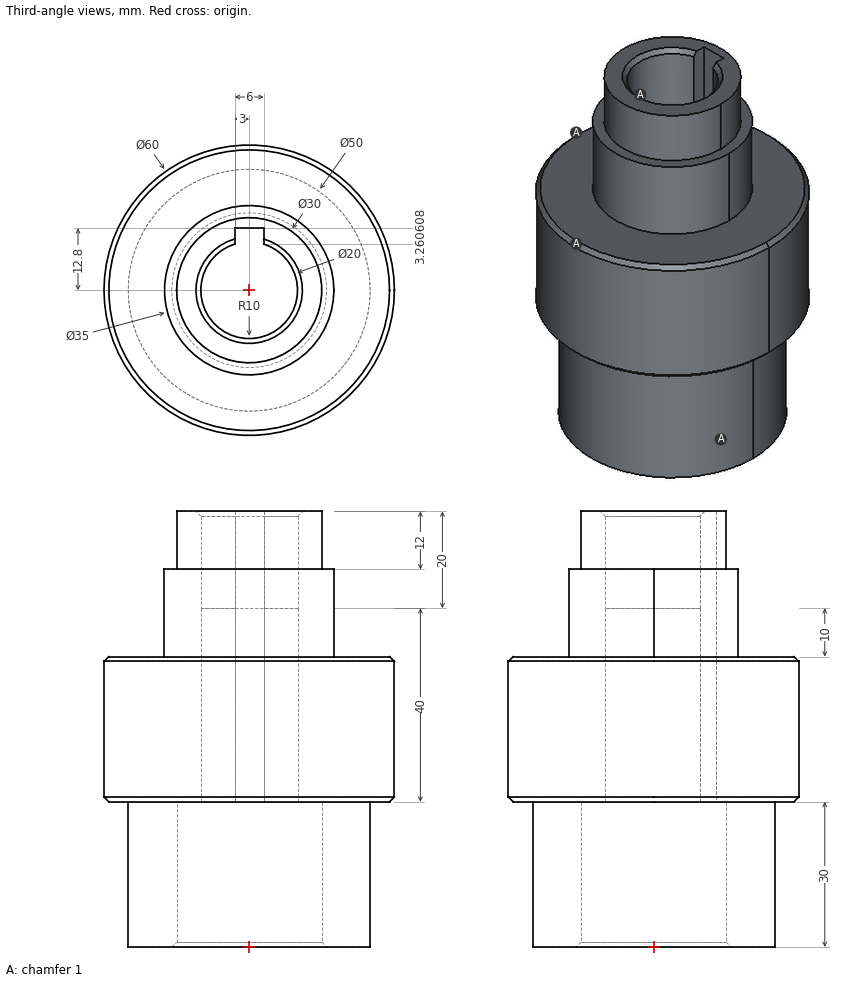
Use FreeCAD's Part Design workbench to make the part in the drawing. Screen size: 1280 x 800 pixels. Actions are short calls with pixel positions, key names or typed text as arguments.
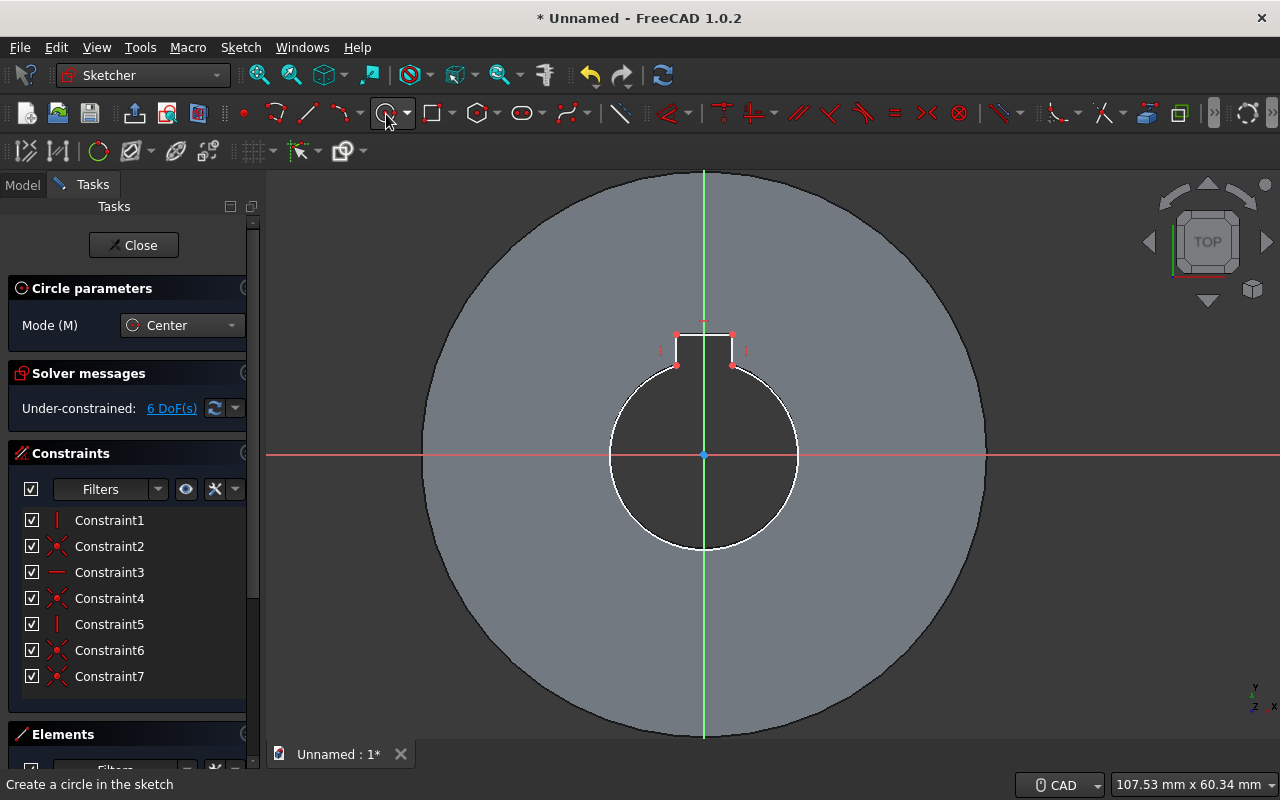
click(704, 454)
move(821, 338)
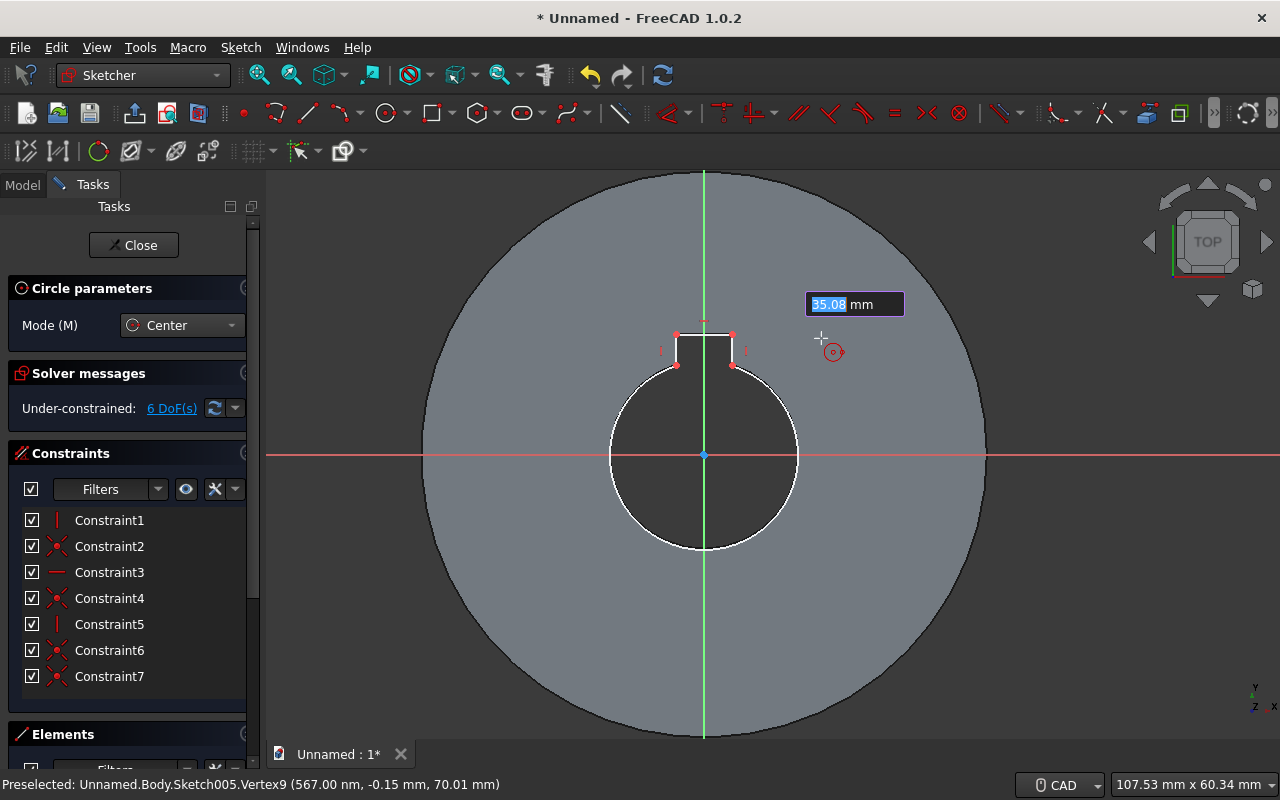
text(35)
key(Return)
key(Escape)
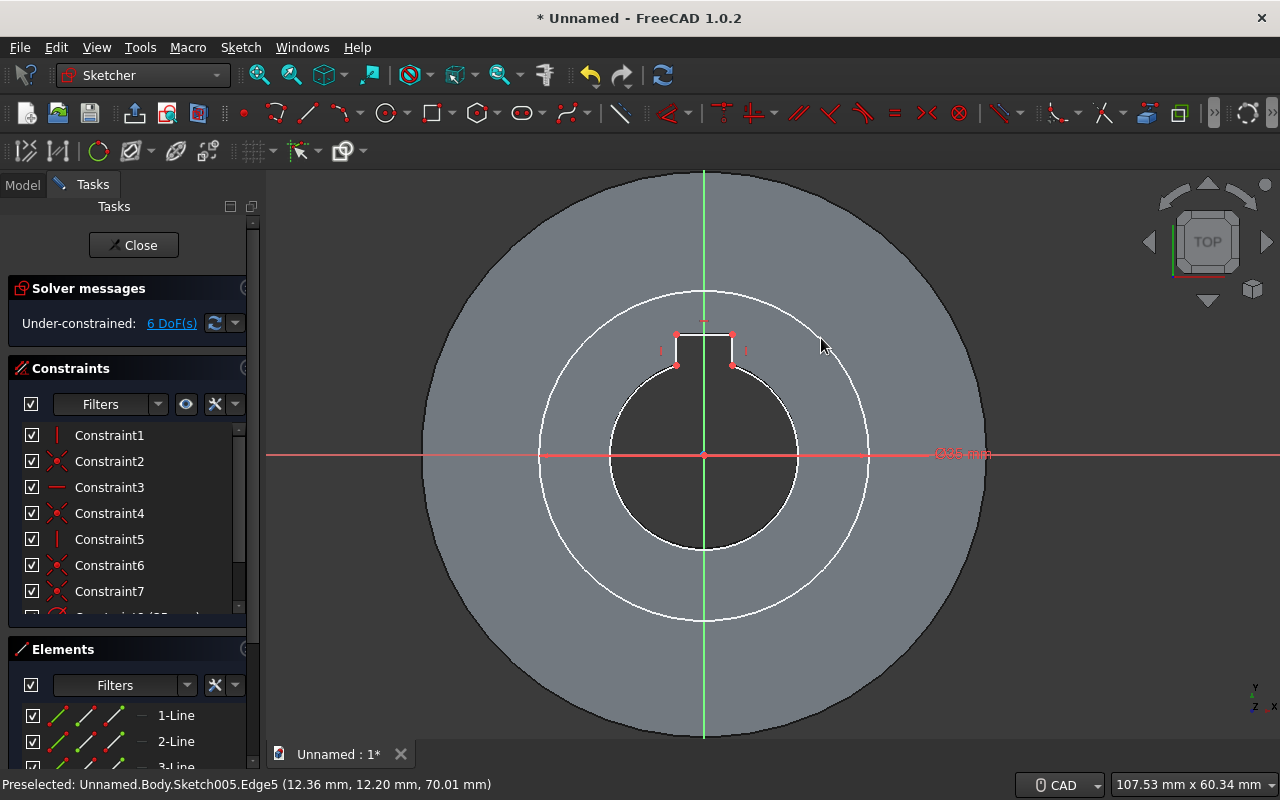
drag(694, 444, 714, 466)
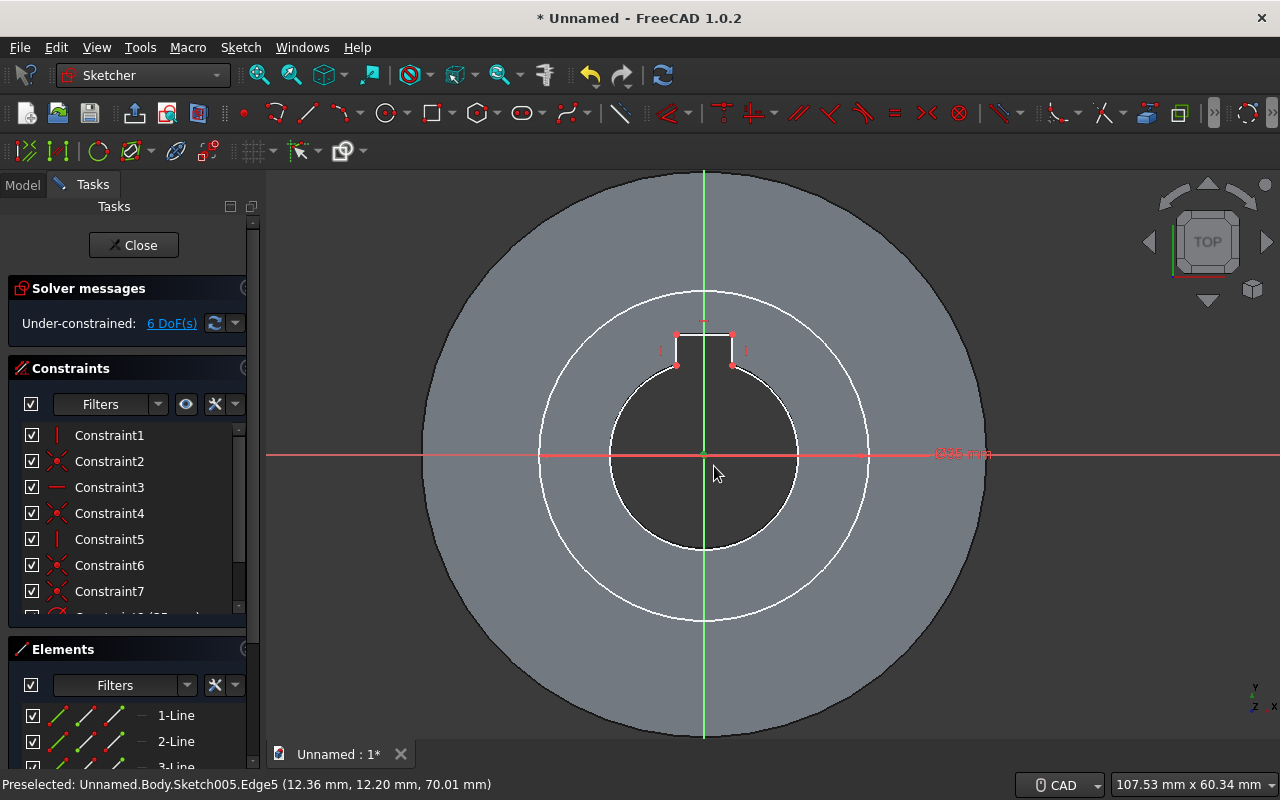
click(722, 114)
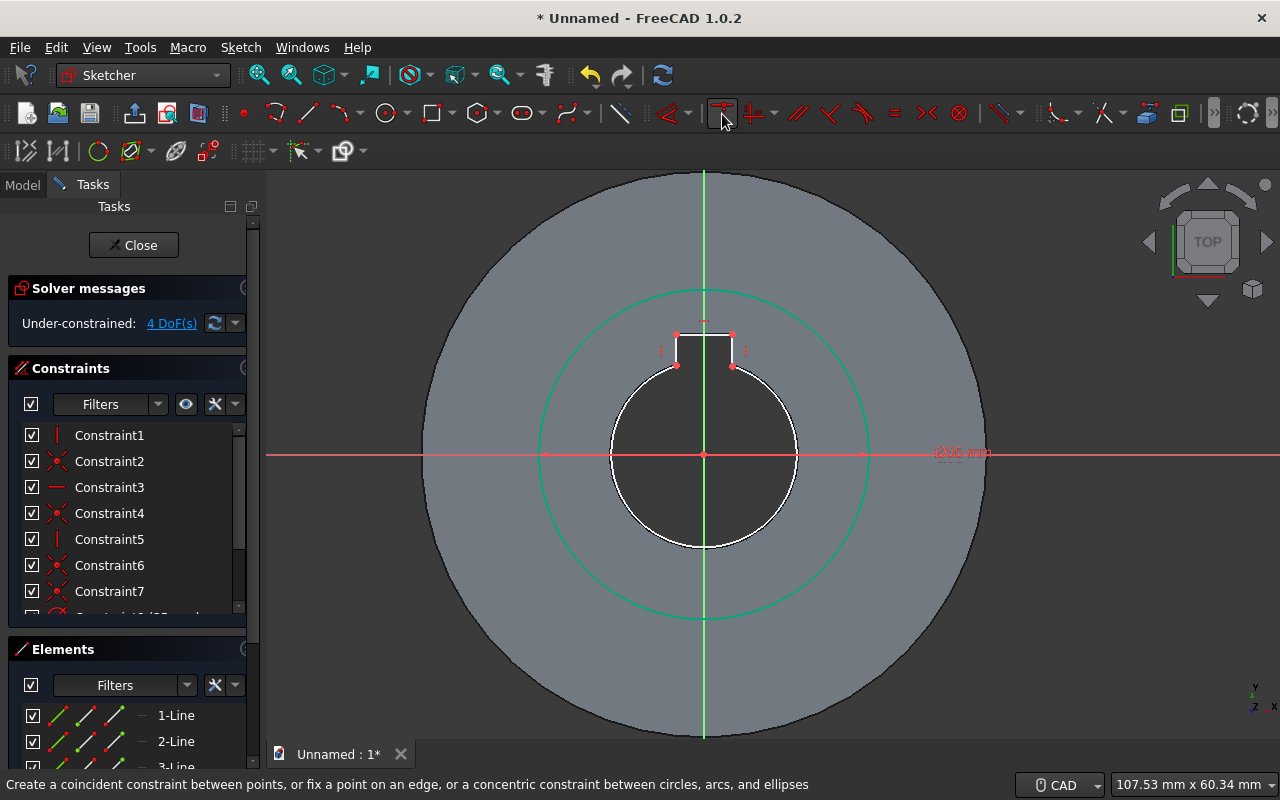
click(668, 114)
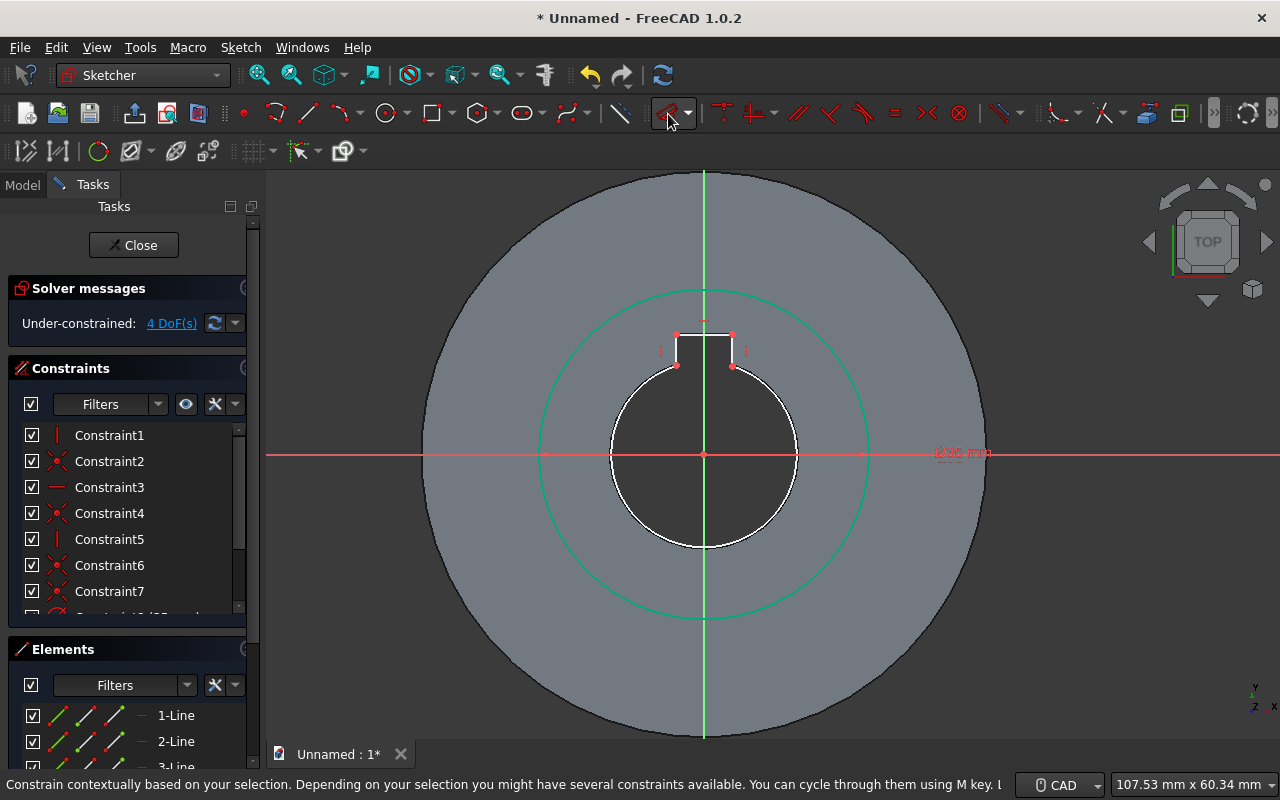
click(620, 494)
click(591, 508)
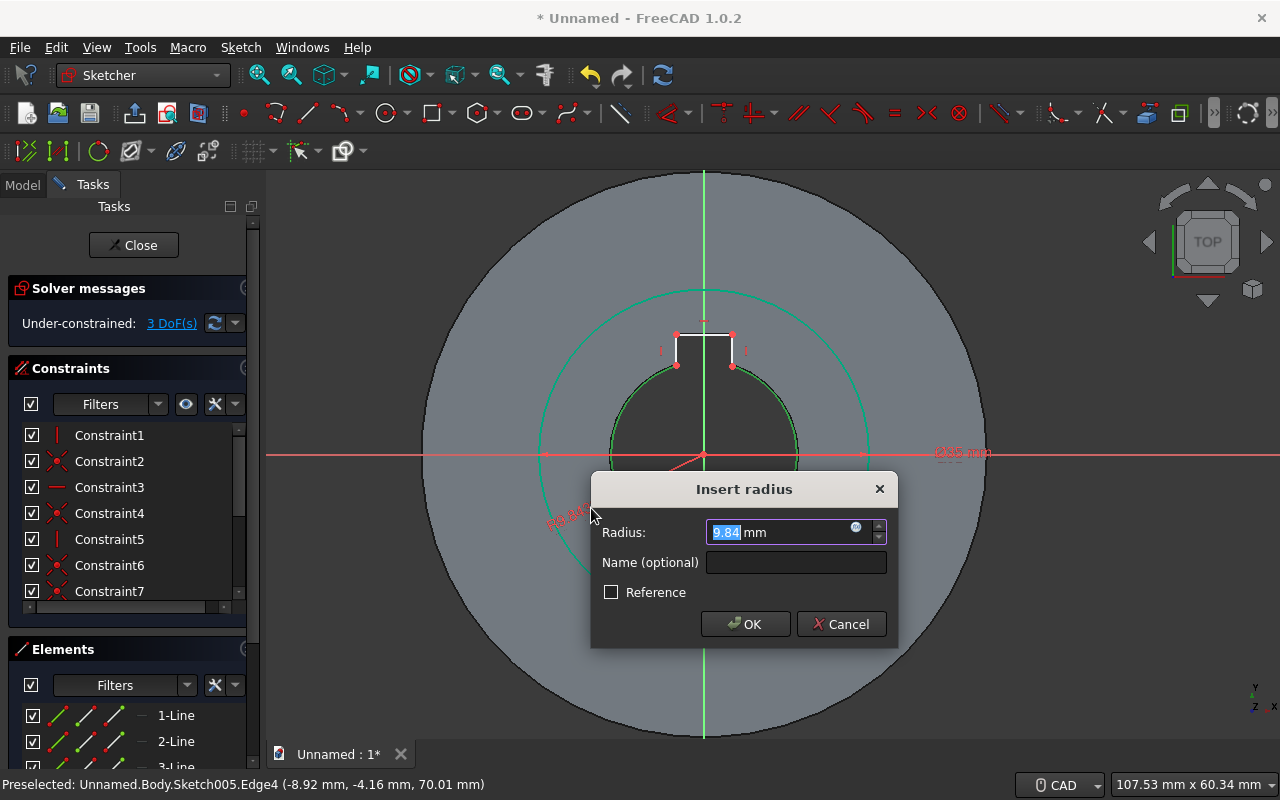
text(10)
key(Return)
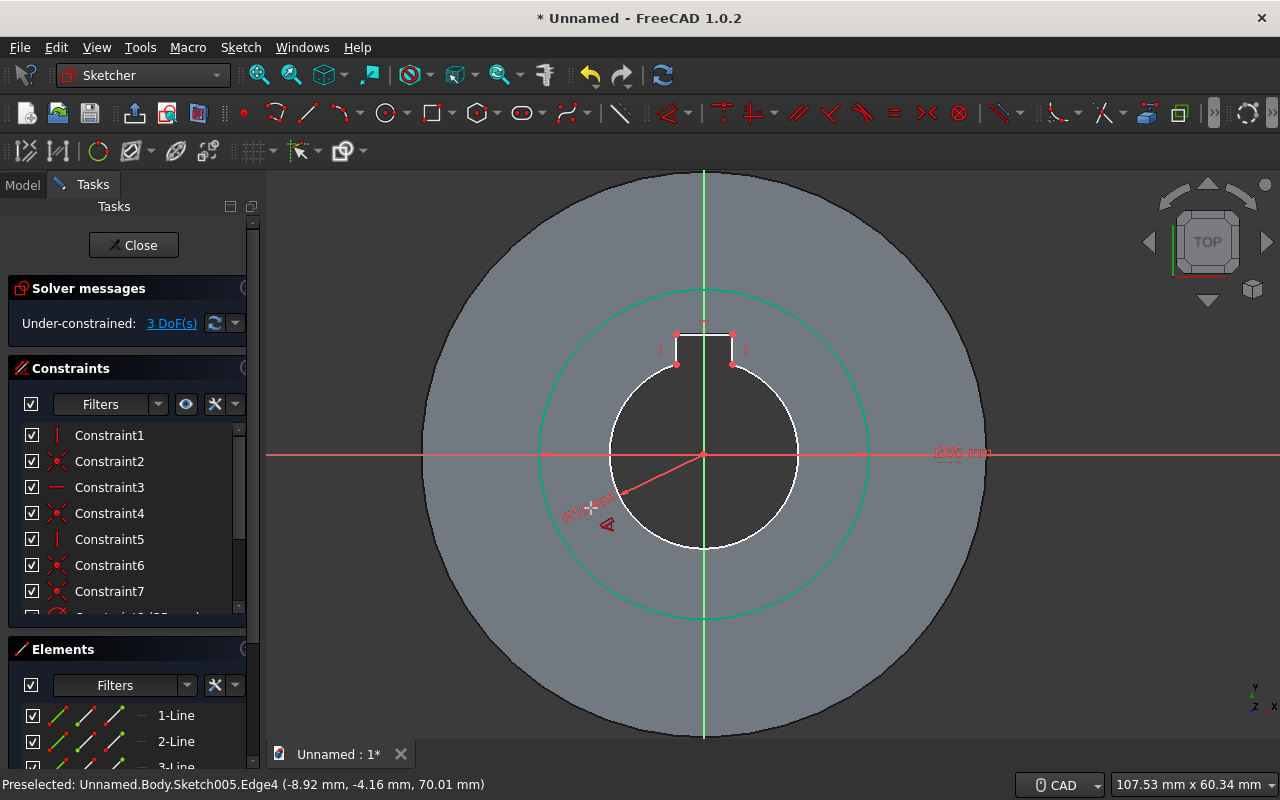
scroll(693, 335, up, 2)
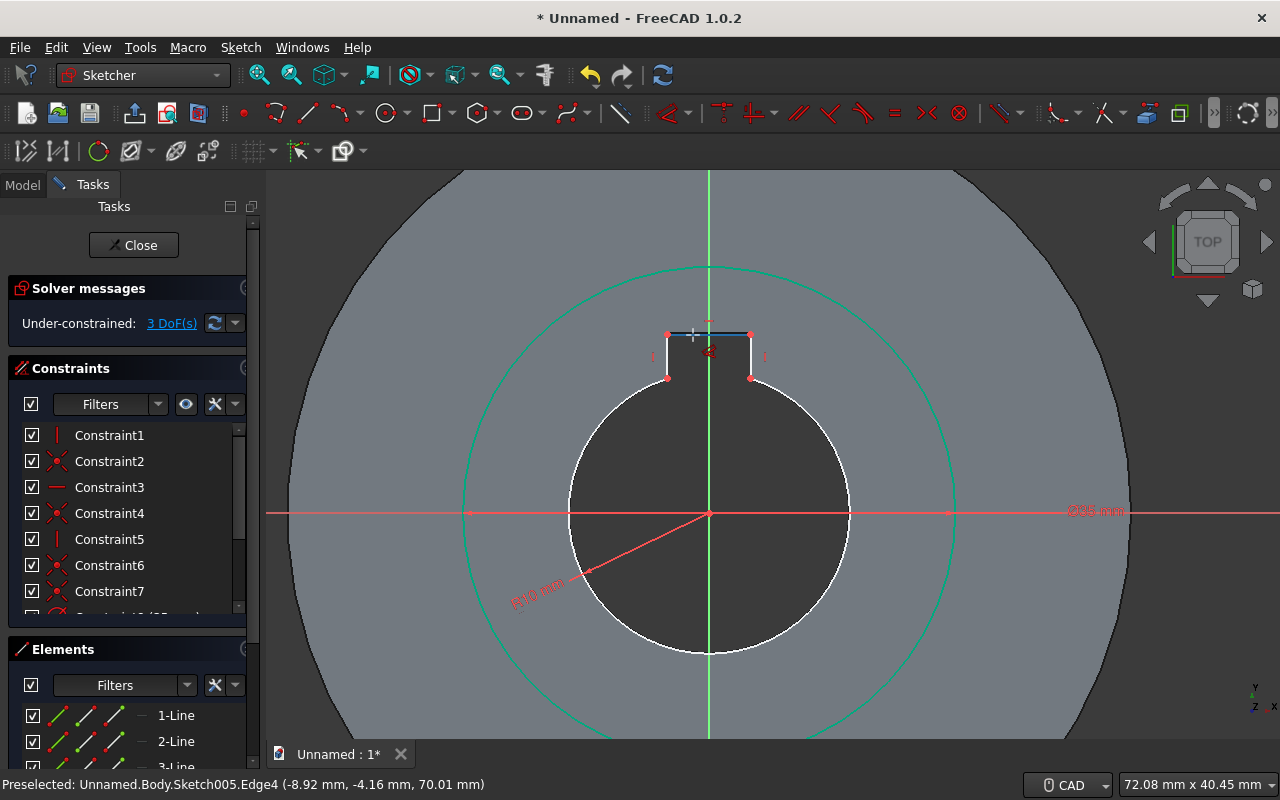
click(692, 335)
click(690, 301)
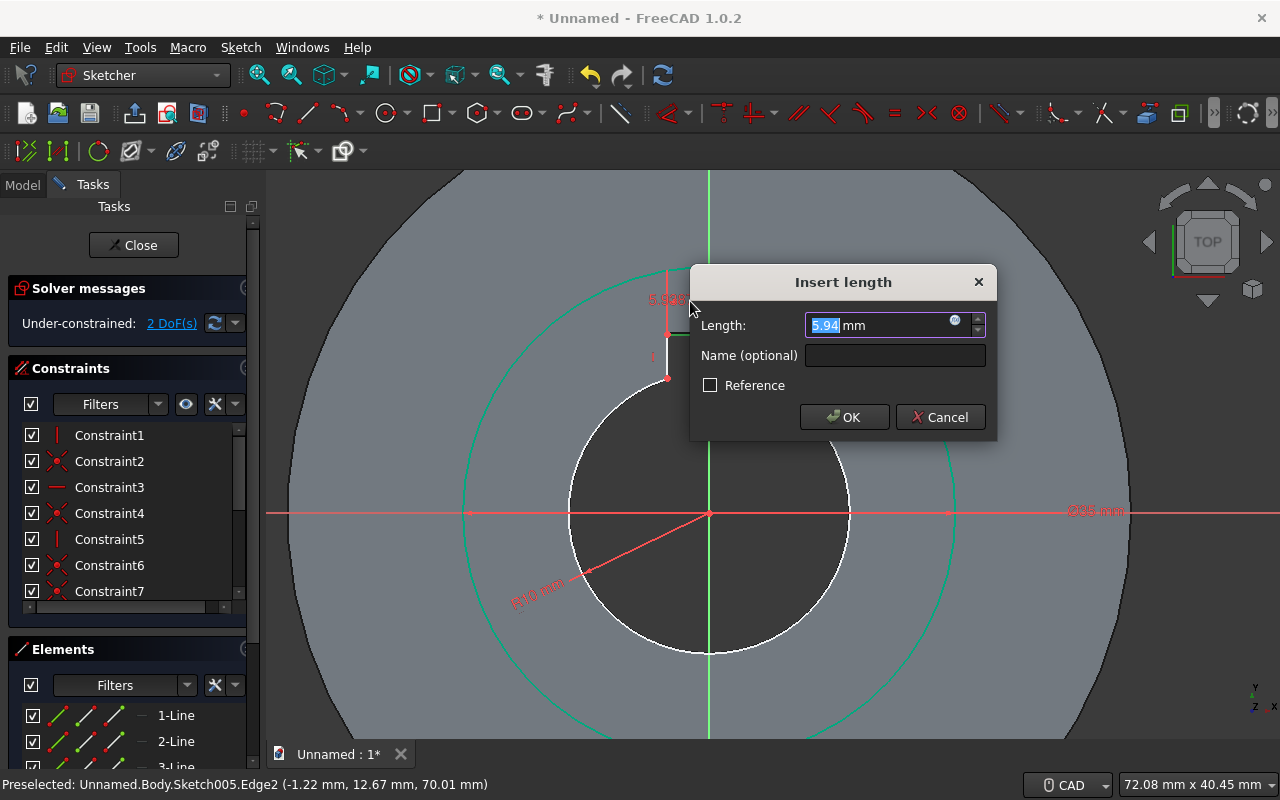
text(6)
key(Return)